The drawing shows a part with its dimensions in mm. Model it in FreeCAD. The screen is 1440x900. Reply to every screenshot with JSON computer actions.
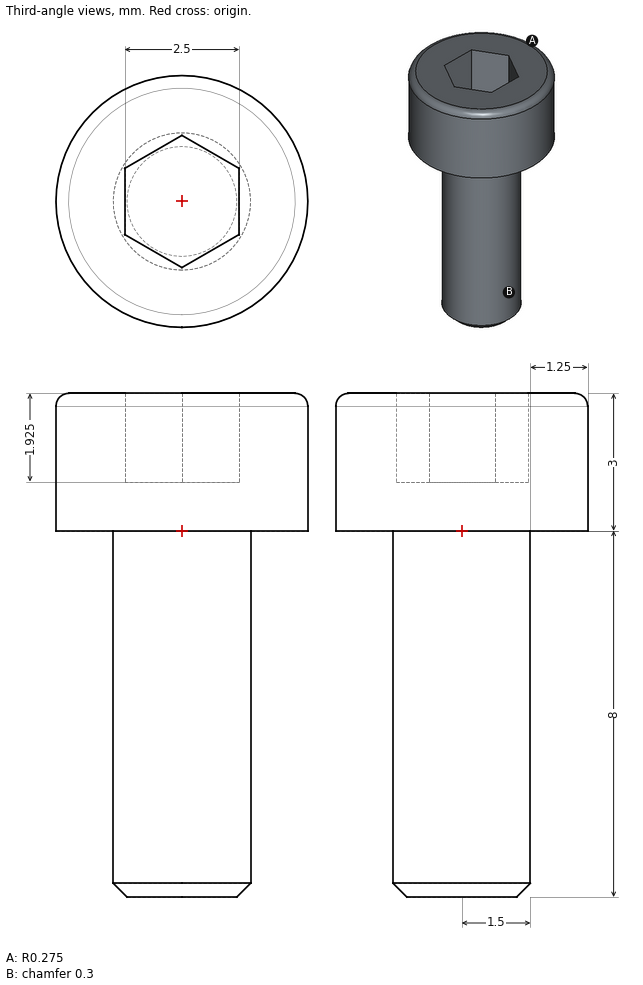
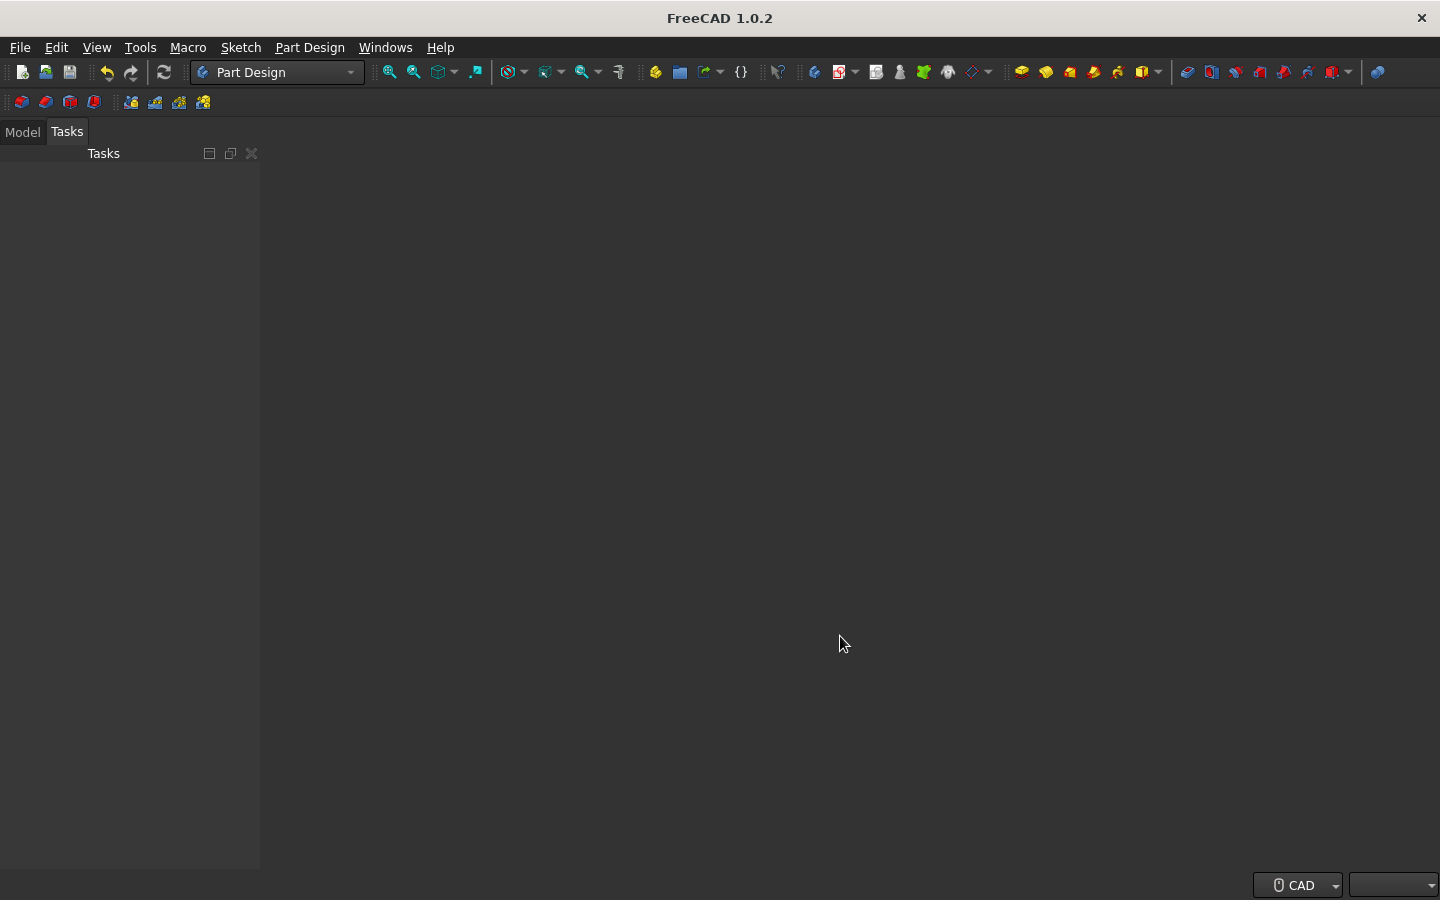
{"action": "left_click", "coordinate": [22, 72]}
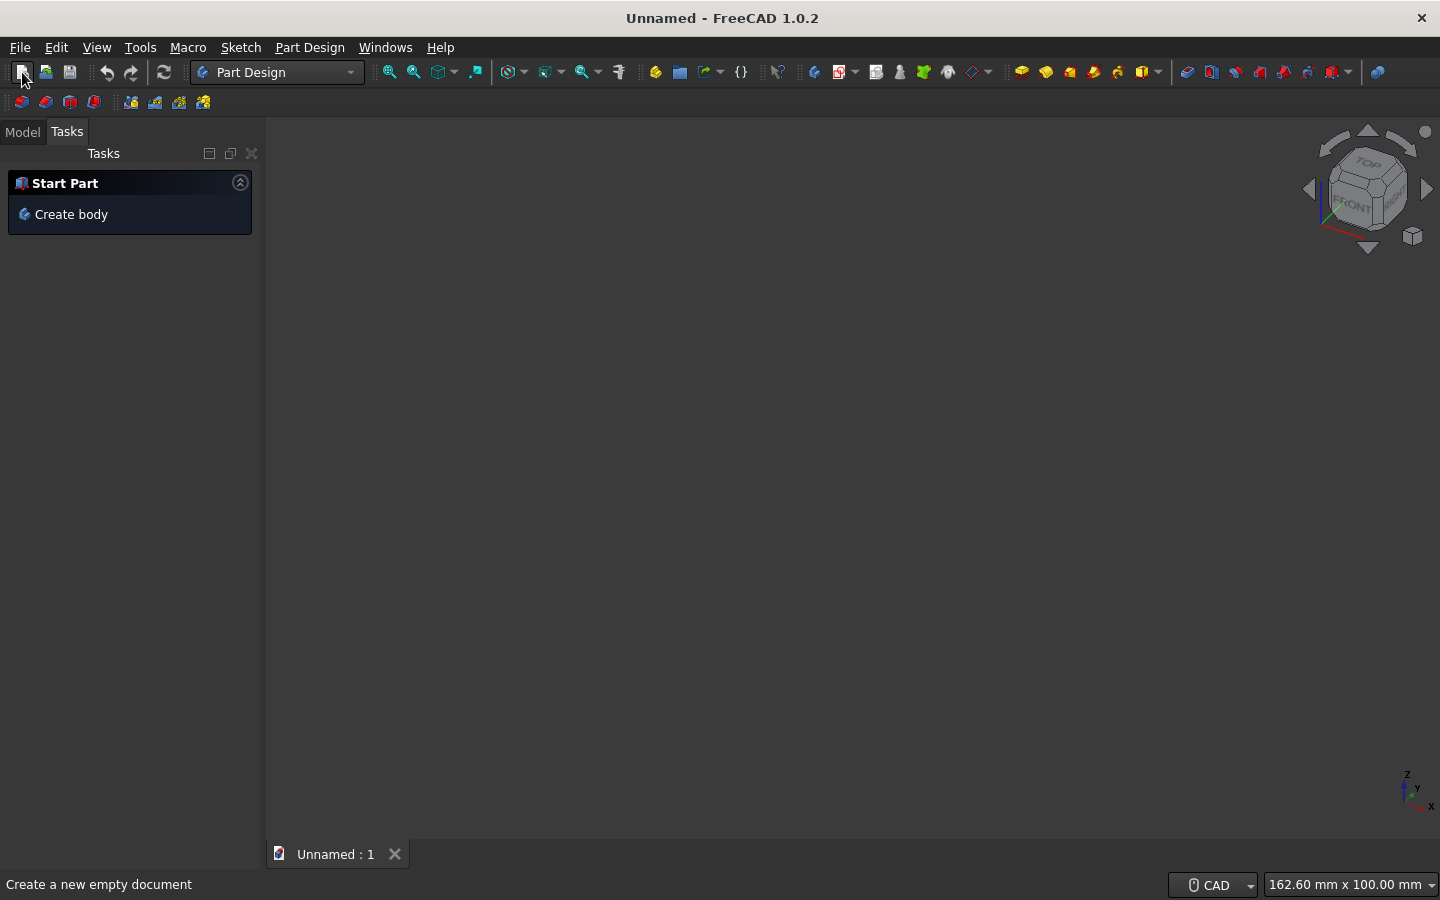
{"action": "left_click", "coordinate": [840, 72]}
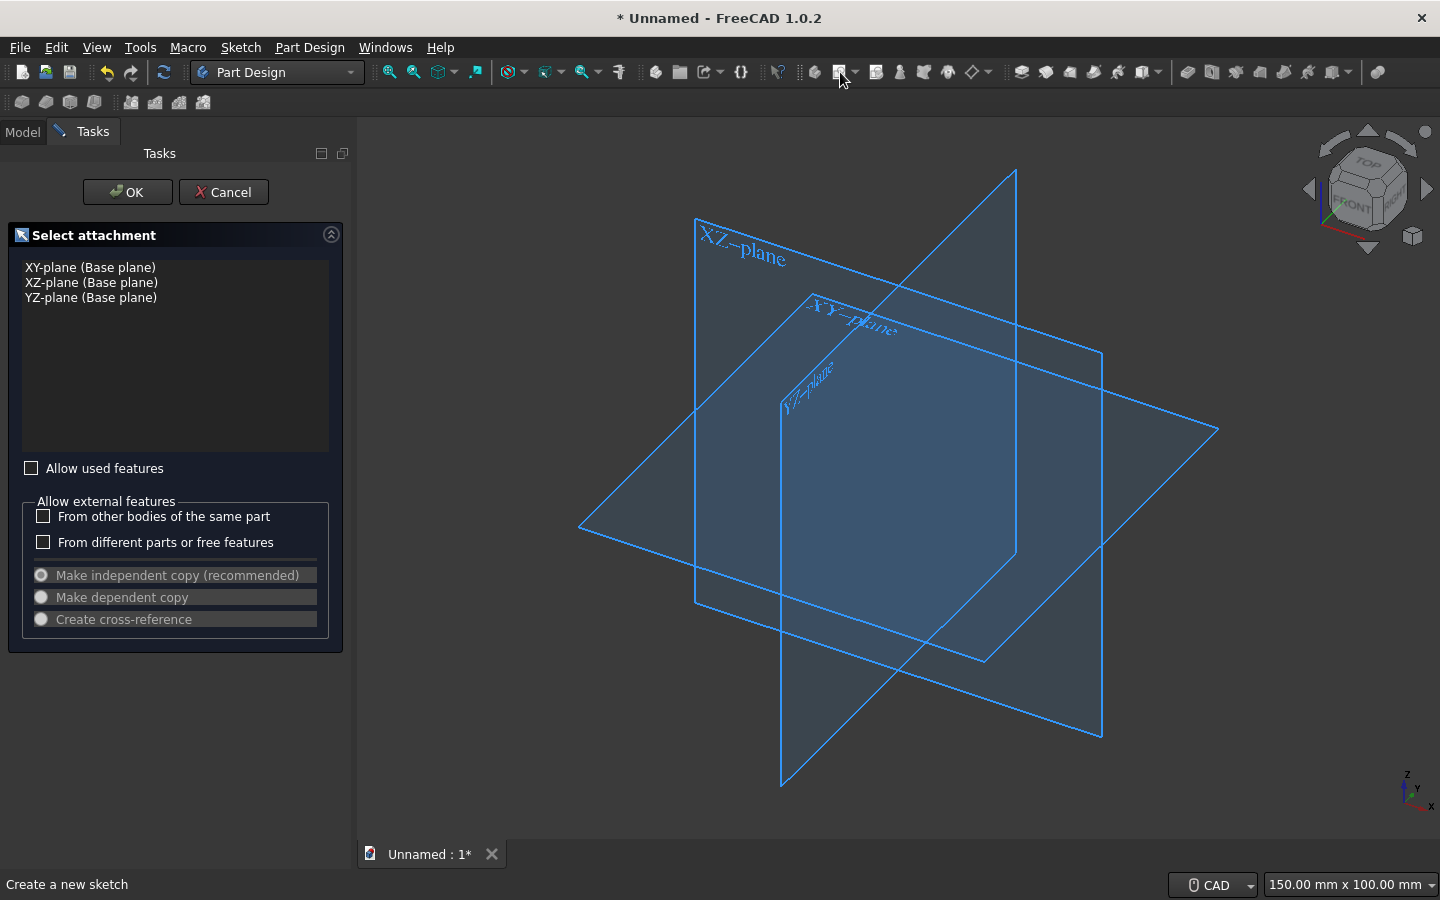
{"action": "left_click", "coordinate": [82, 298]}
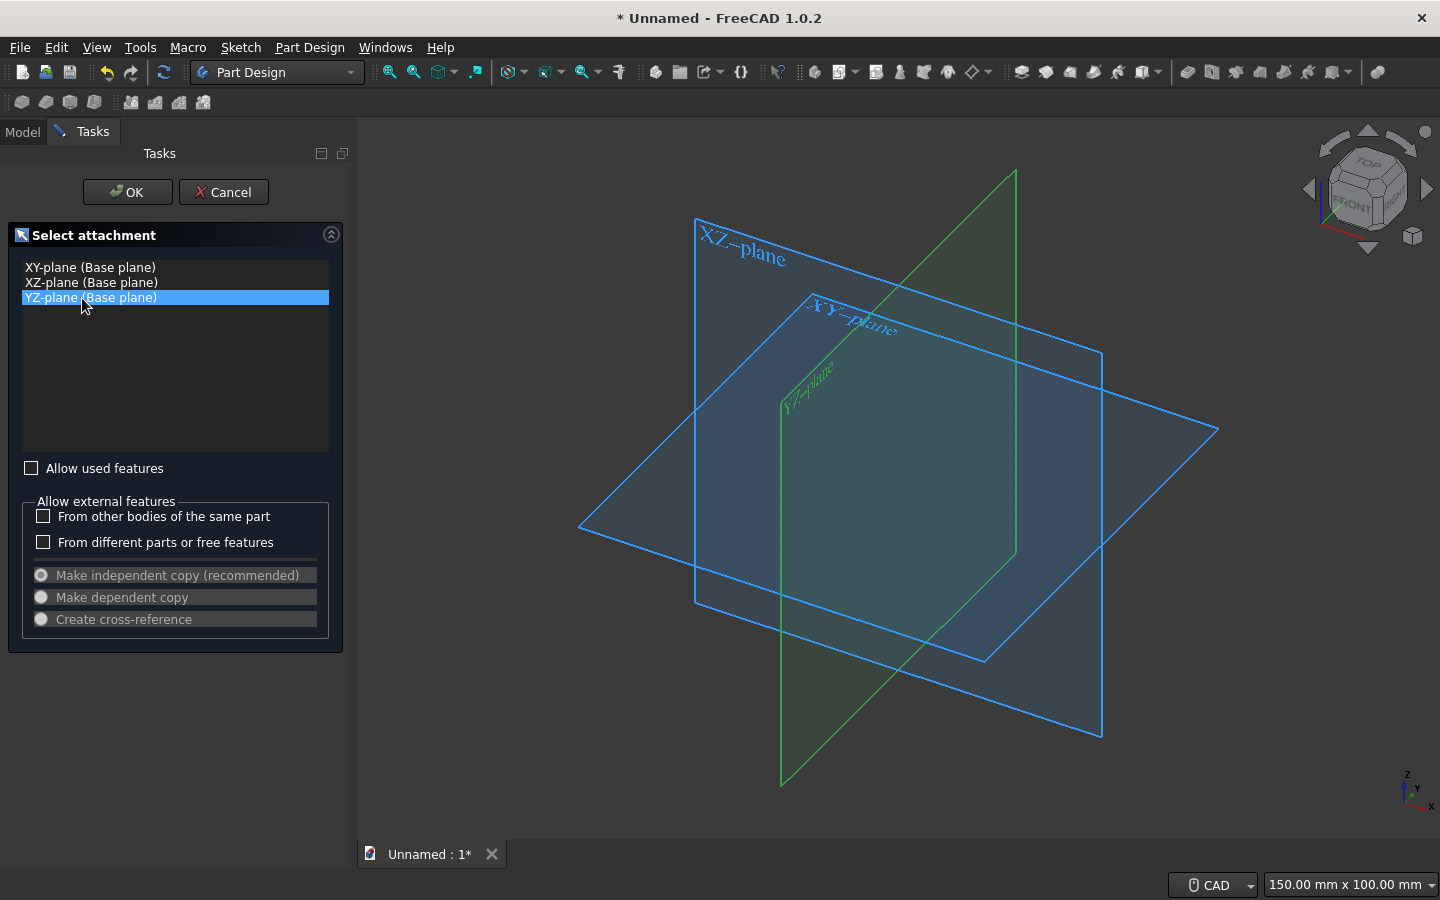
{"action": "left_click", "coordinate": [128, 192]}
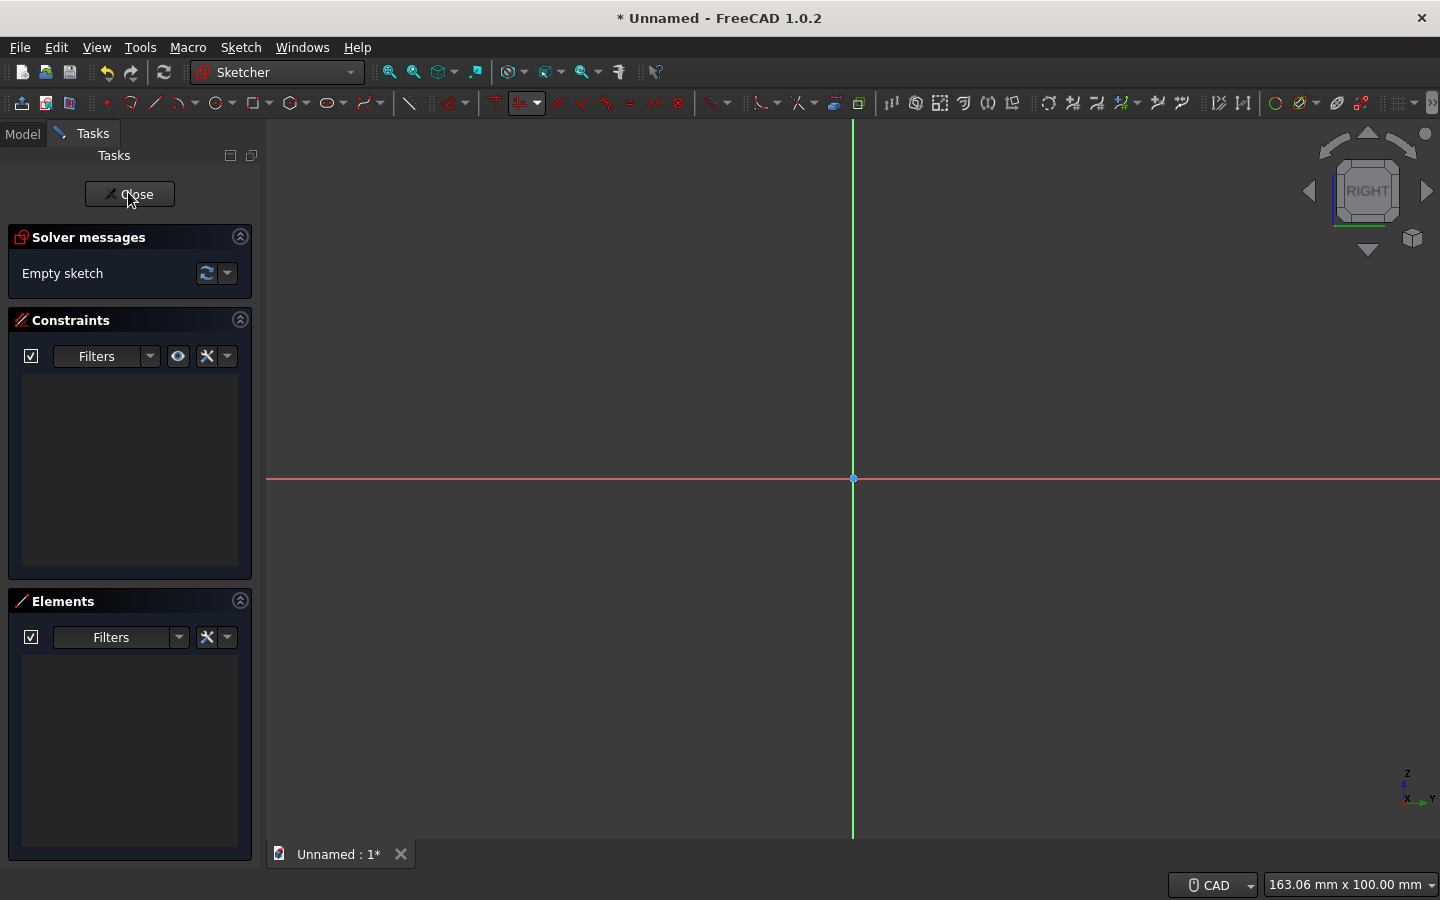
{"action": "scroll", "coordinate": [878, 501], "scroll_direction": "up", "scroll_amount": 9}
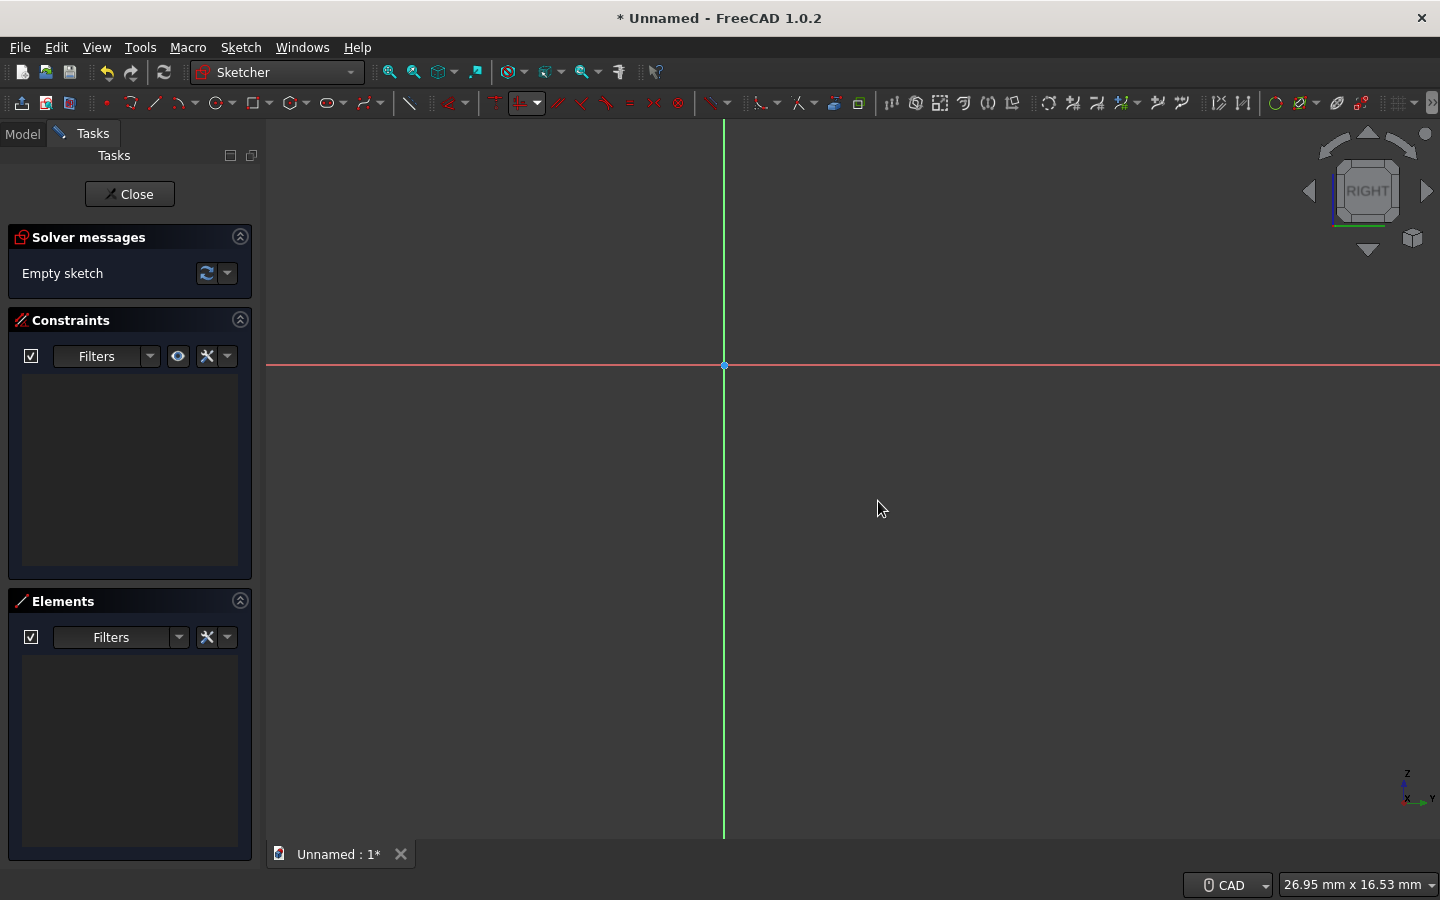
{"action": "left_click", "coordinate": [132, 104]}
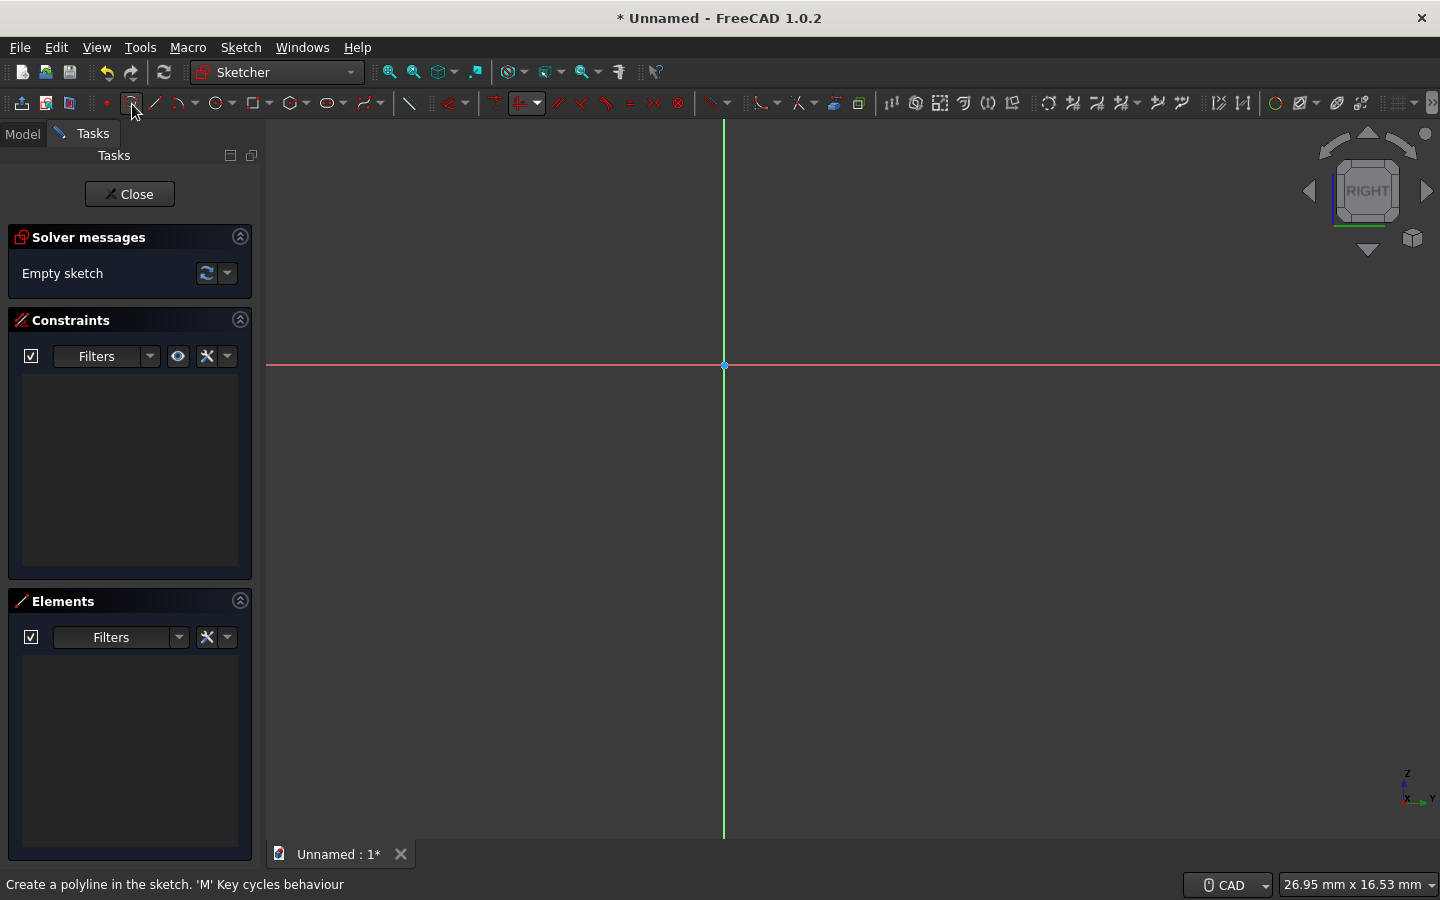
{"action": "left_click", "coordinate": [789, 365]}
{"action": "left_click", "coordinate": [844, 374]}
{"action": "left_click", "coordinate": [844, 235]}
{"action": "left_click", "coordinate": [724, 235]}
{"action": "left_click", "coordinate": [733, 714]}
{"action": "left_click", "coordinate": [789, 714]}
{"action": "left_click", "coordinate": [789, 365]}
{"action": "key", "text": "Escape"}
{"action": "key", "text": "Escape"}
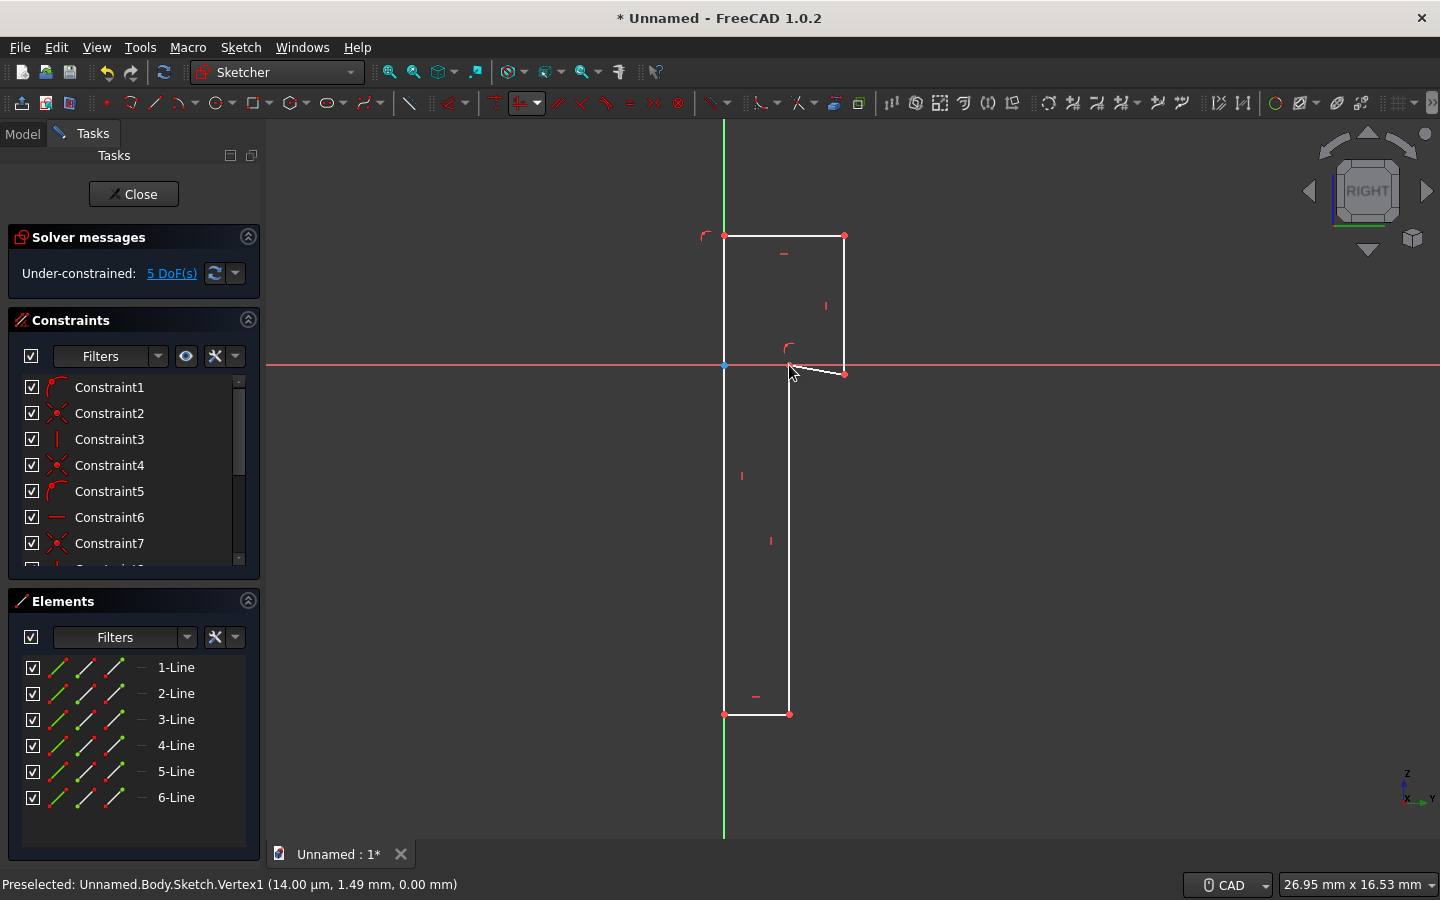
{"action": "left_click", "coordinate": [805, 368]}